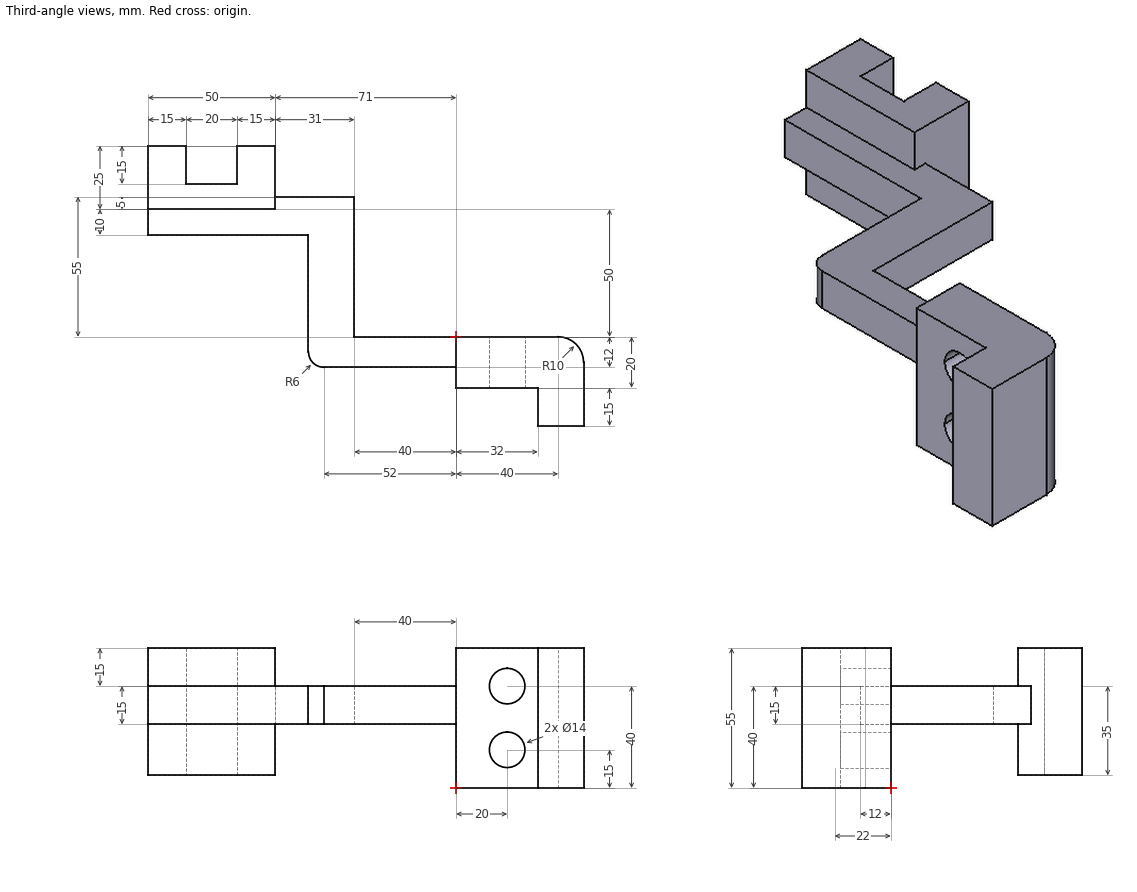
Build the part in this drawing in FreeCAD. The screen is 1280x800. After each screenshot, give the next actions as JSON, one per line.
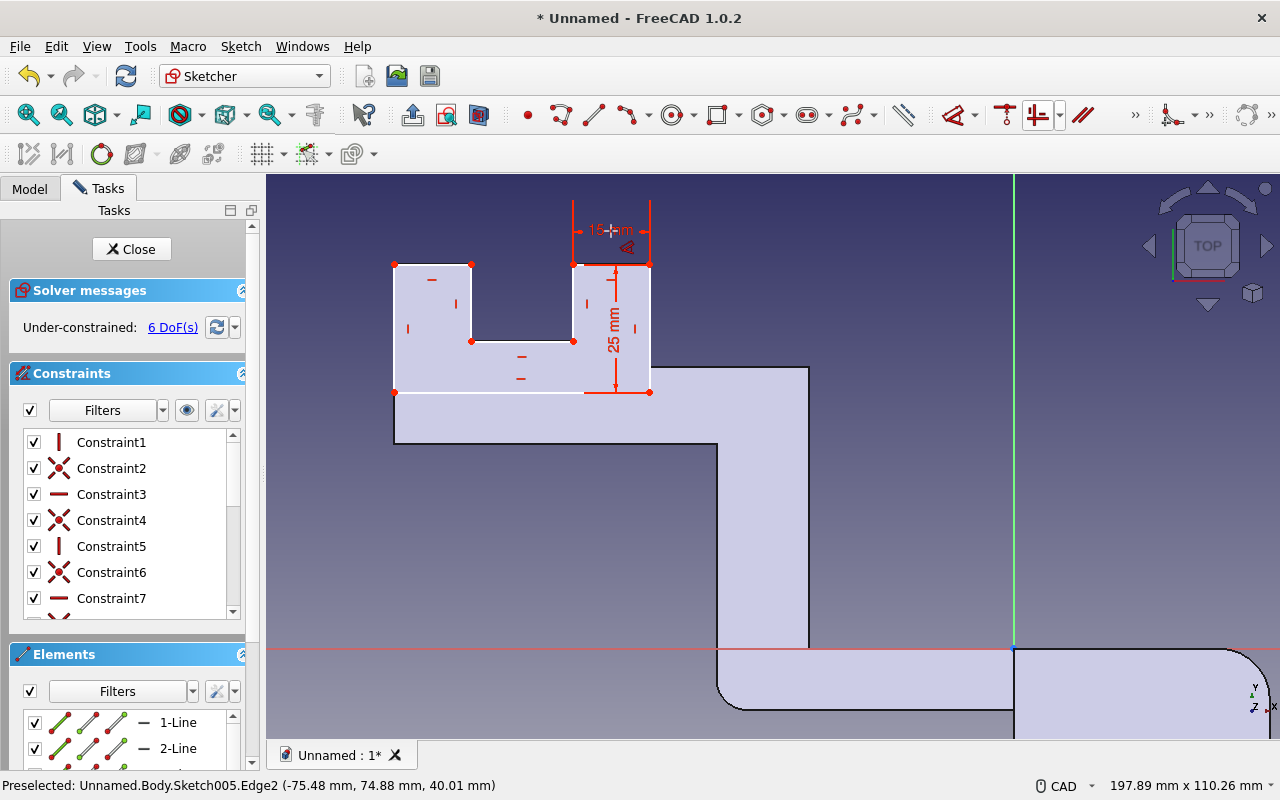
{"action": "left_click", "coordinate": [573, 288]}
{"action": "left_click", "coordinate": [539, 303]}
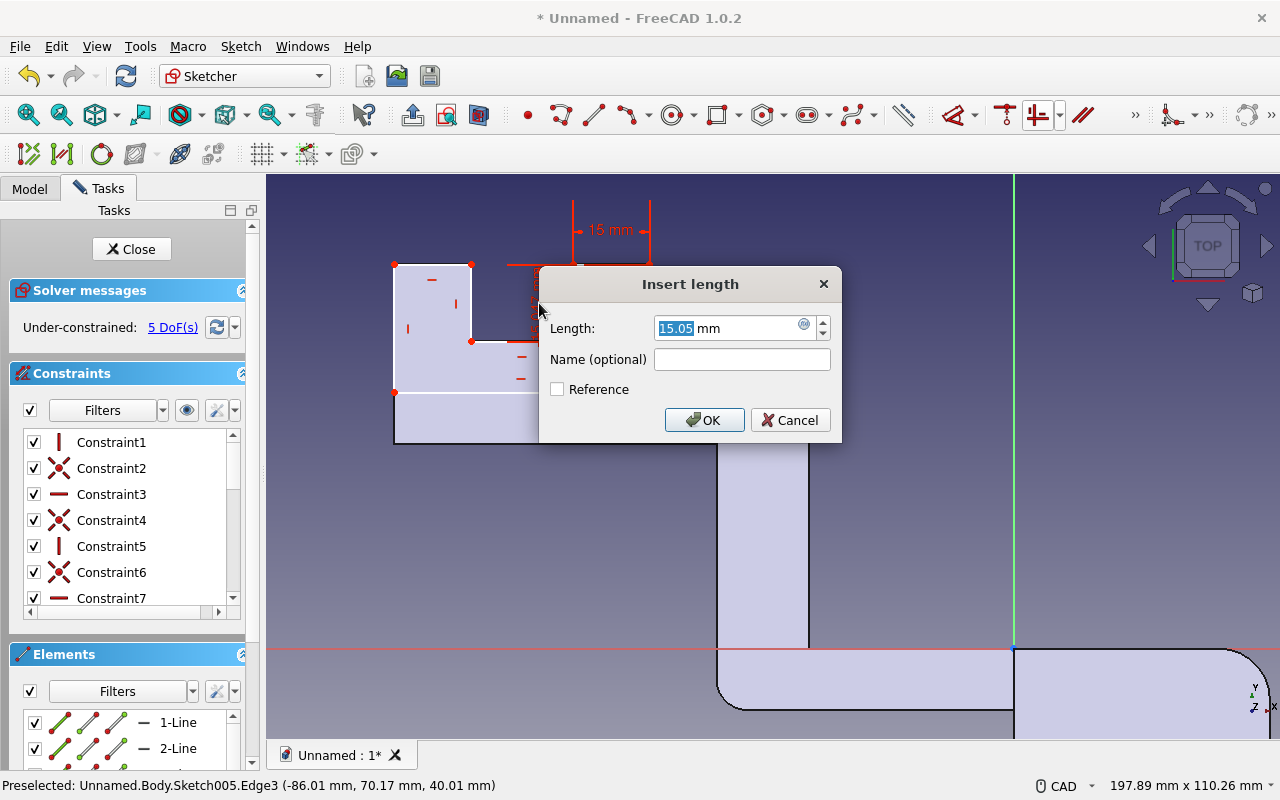
{"action": "type", "text": "15"}
{"action": "key", "text": "Return"}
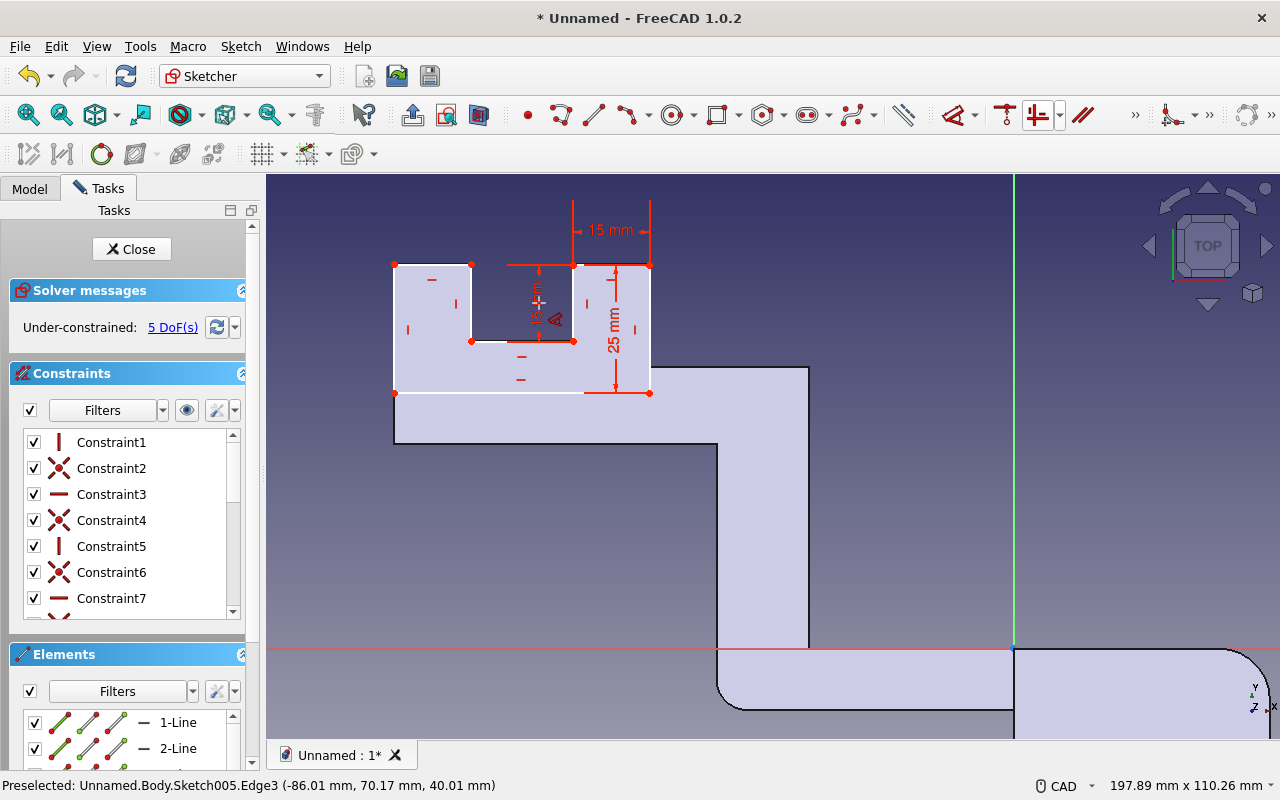
{"action": "left_click", "coordinate": [542, 342]}
{"action": "left_click", "coordinate": [522, 376]}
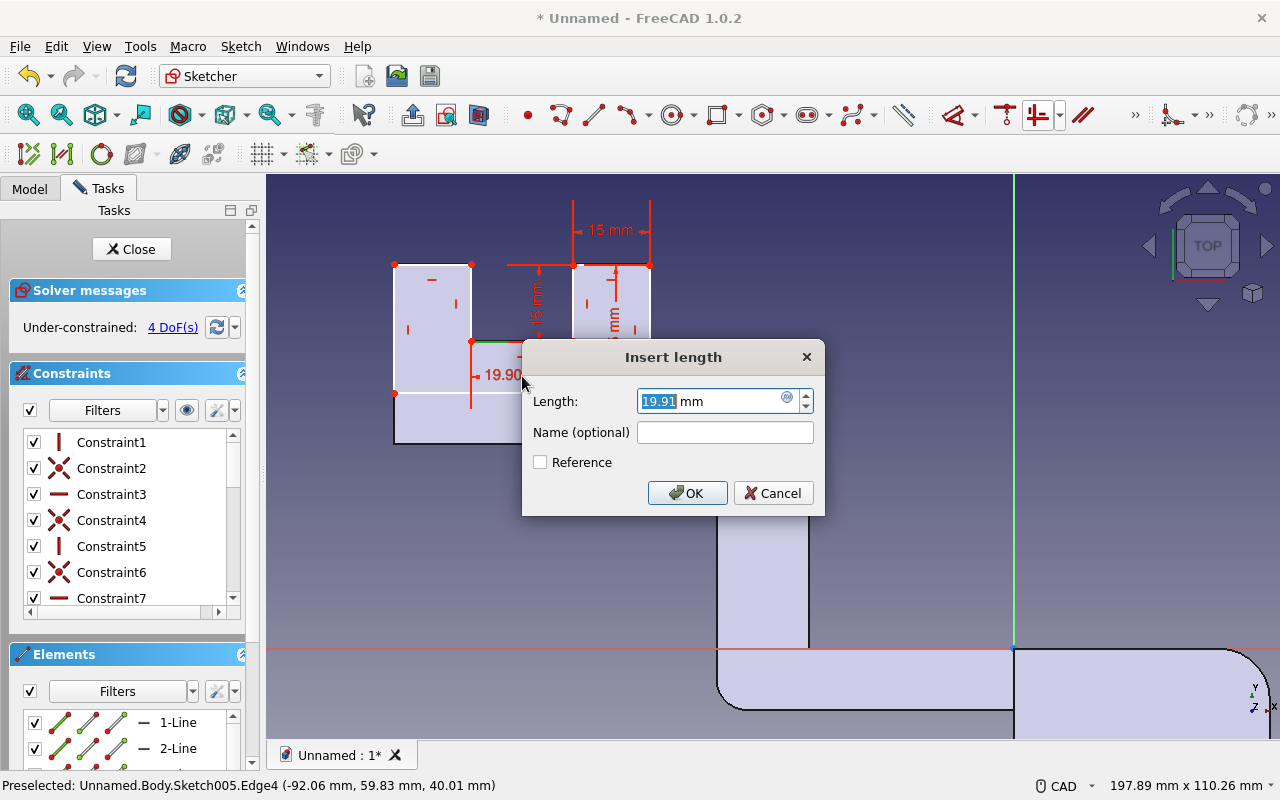
{"action": "type", "text": "20"}
{"action": "key", "text": "Return"}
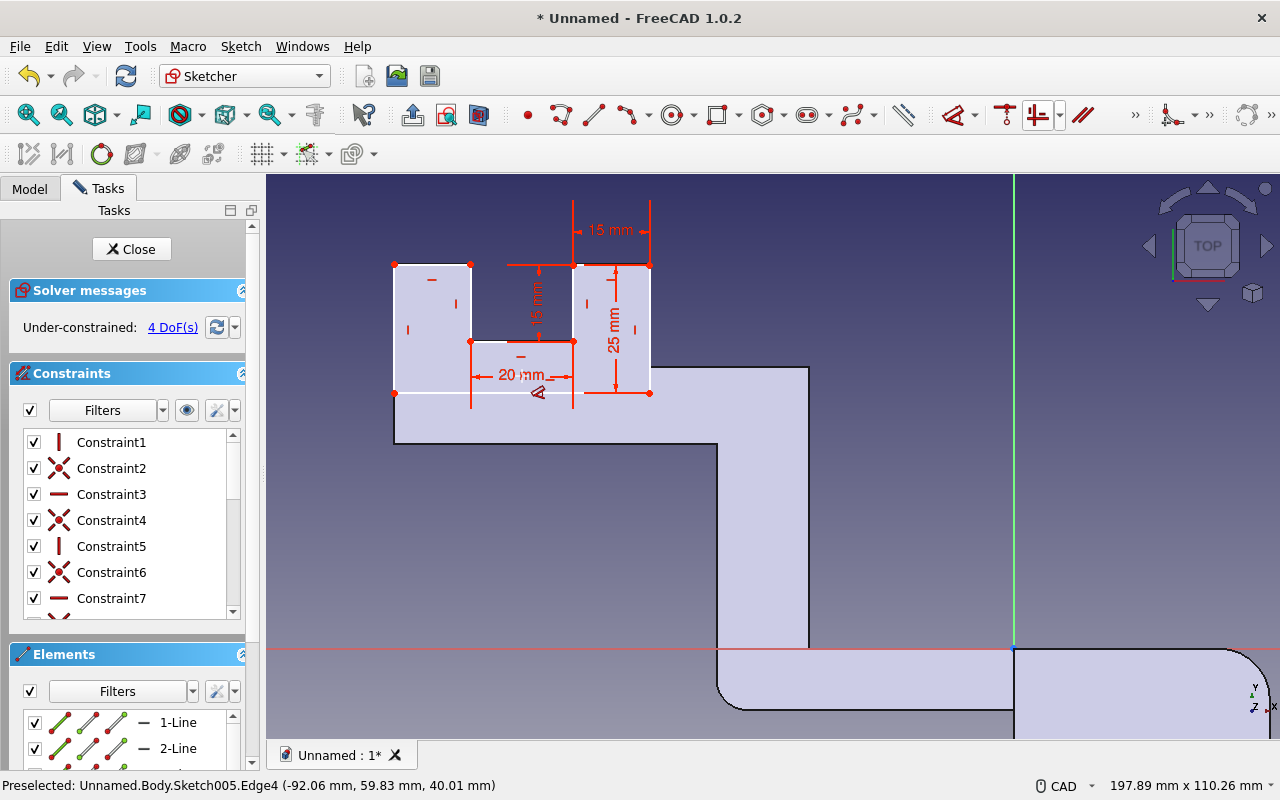
{"action": "left_click", "coordinate": [471, 319]}
{"action": "left_click", "coordinate": [437, 304]}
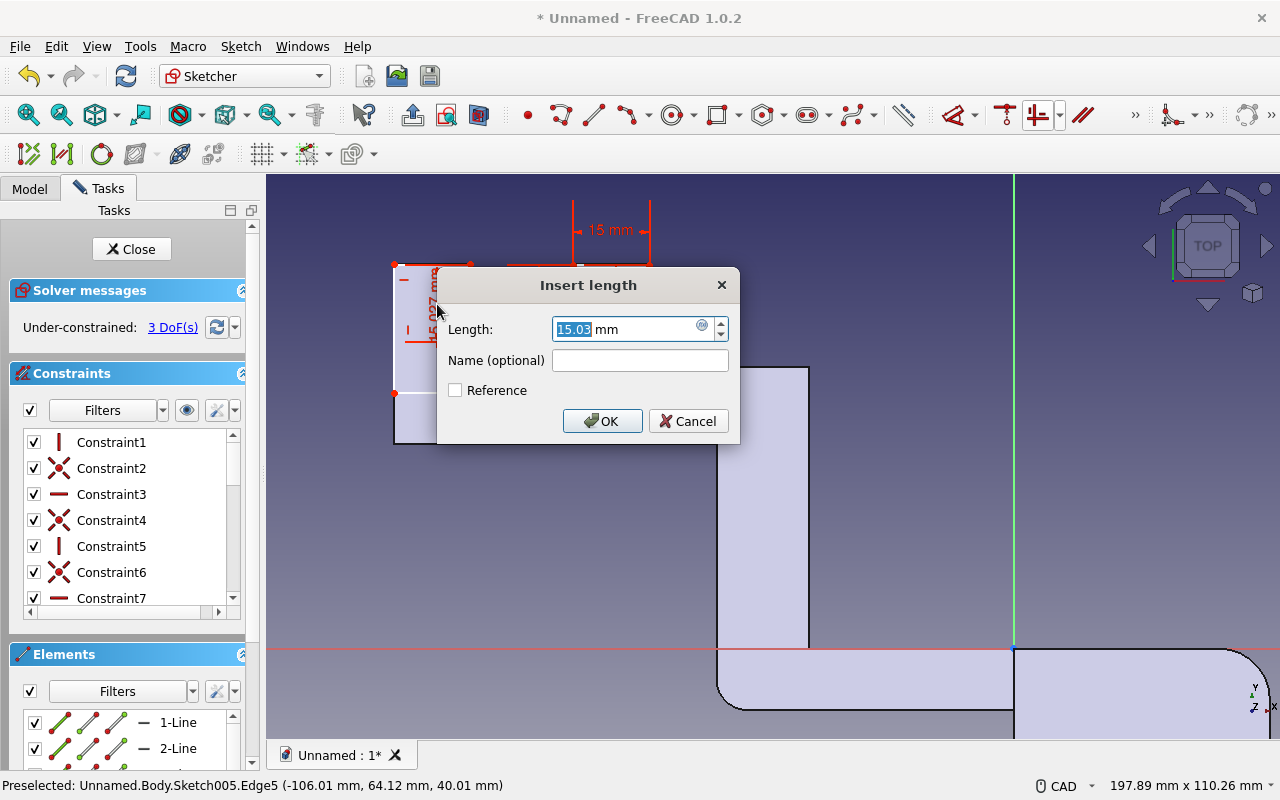
{"action": "type", "text": "15"}
{"action": "key", "text": "Return"}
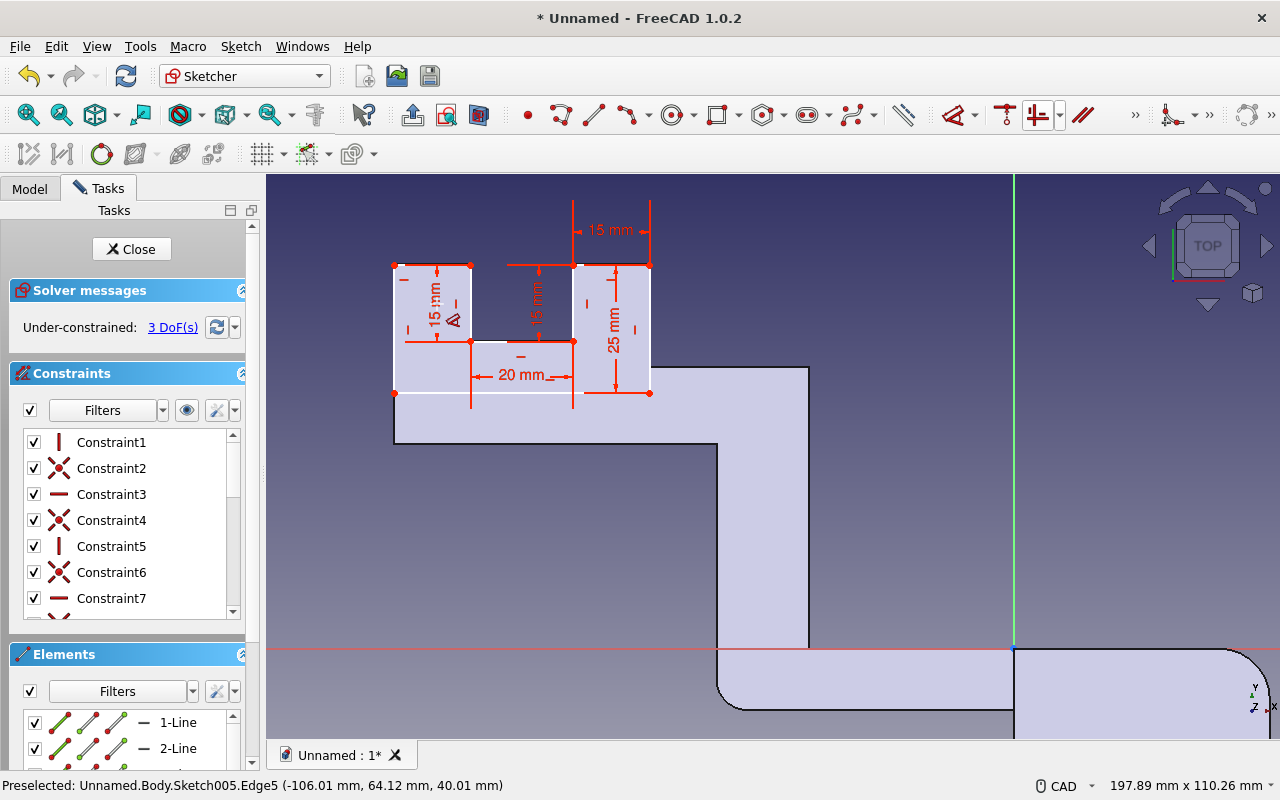
{"action": "left_click", "coordinate": [448, 265]}
{"action": "left_click", "coordinate": [432, 231]}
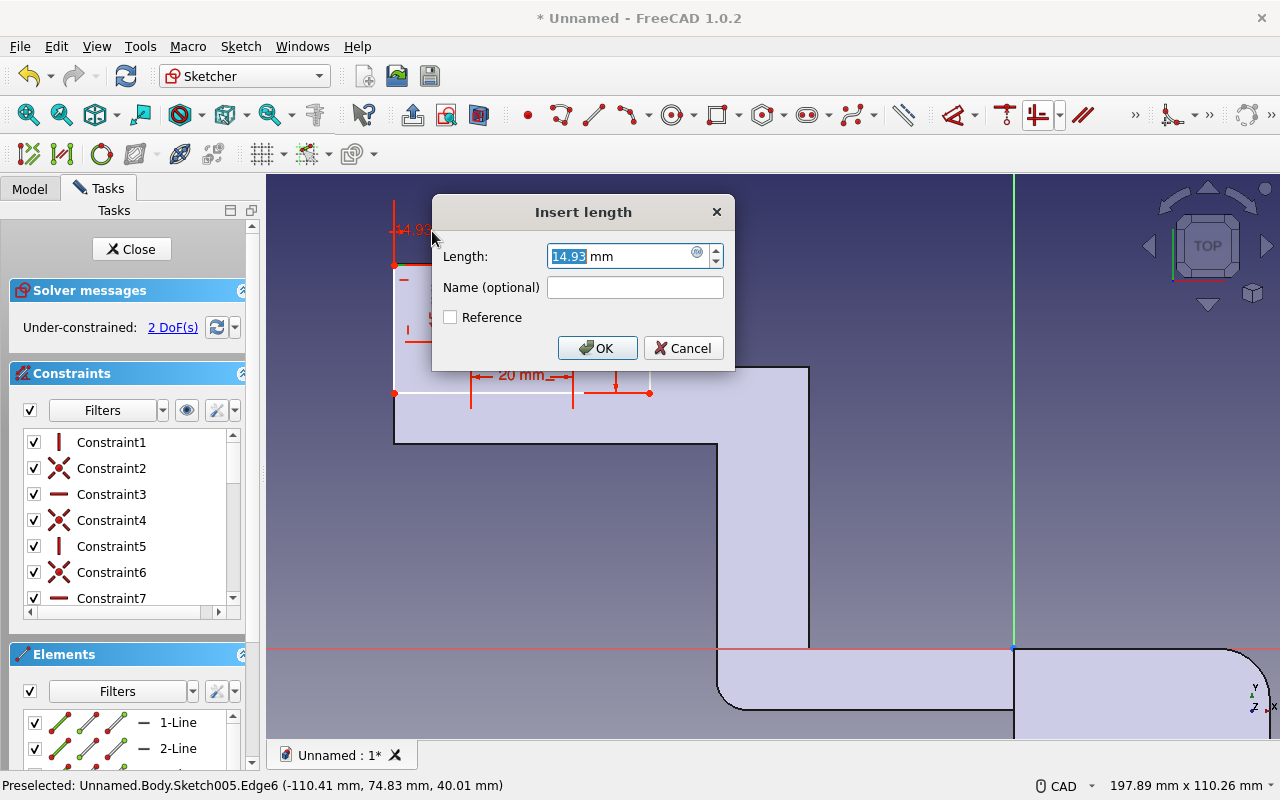
{"action": "type", "text": "15"}
{"action": "key", "text": "Return"}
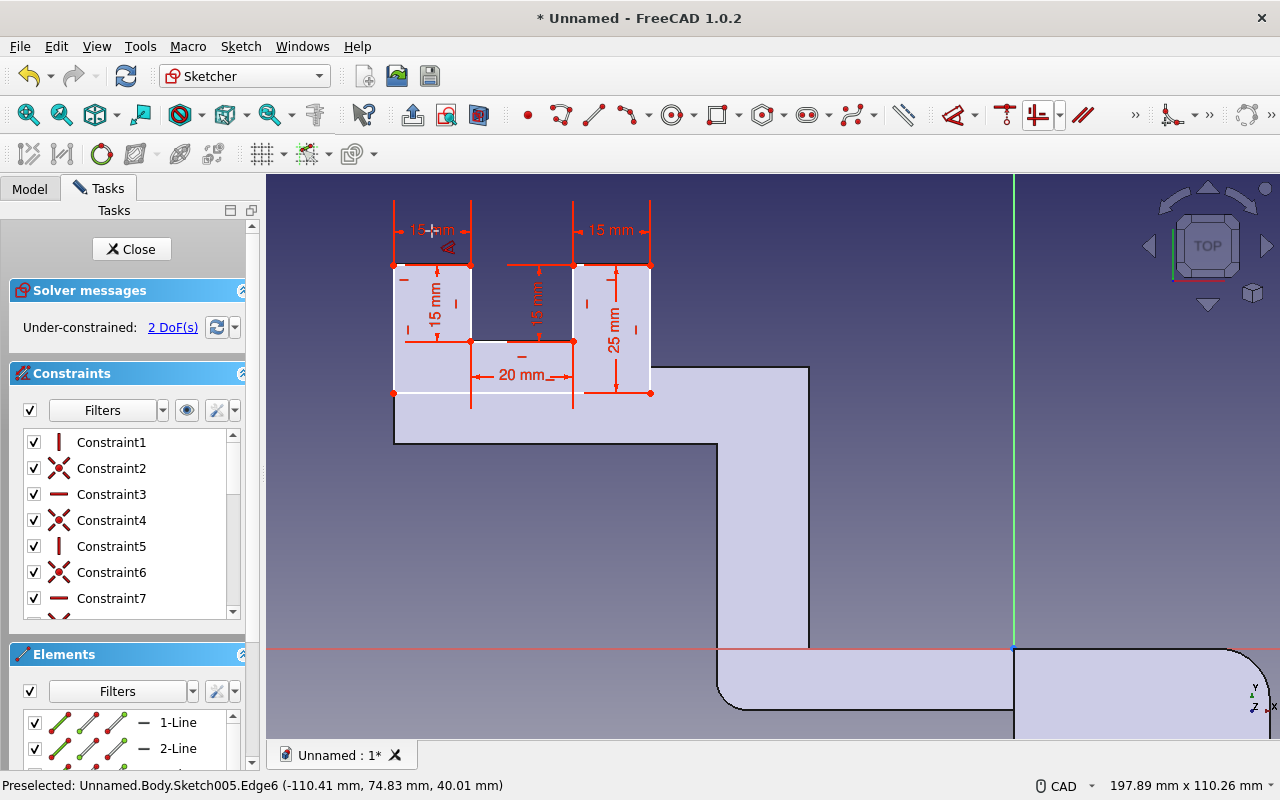
{"action": "left_click", "coordinate": [650, 393]}
{"action": "left_click", "coordinate": [832, 683]}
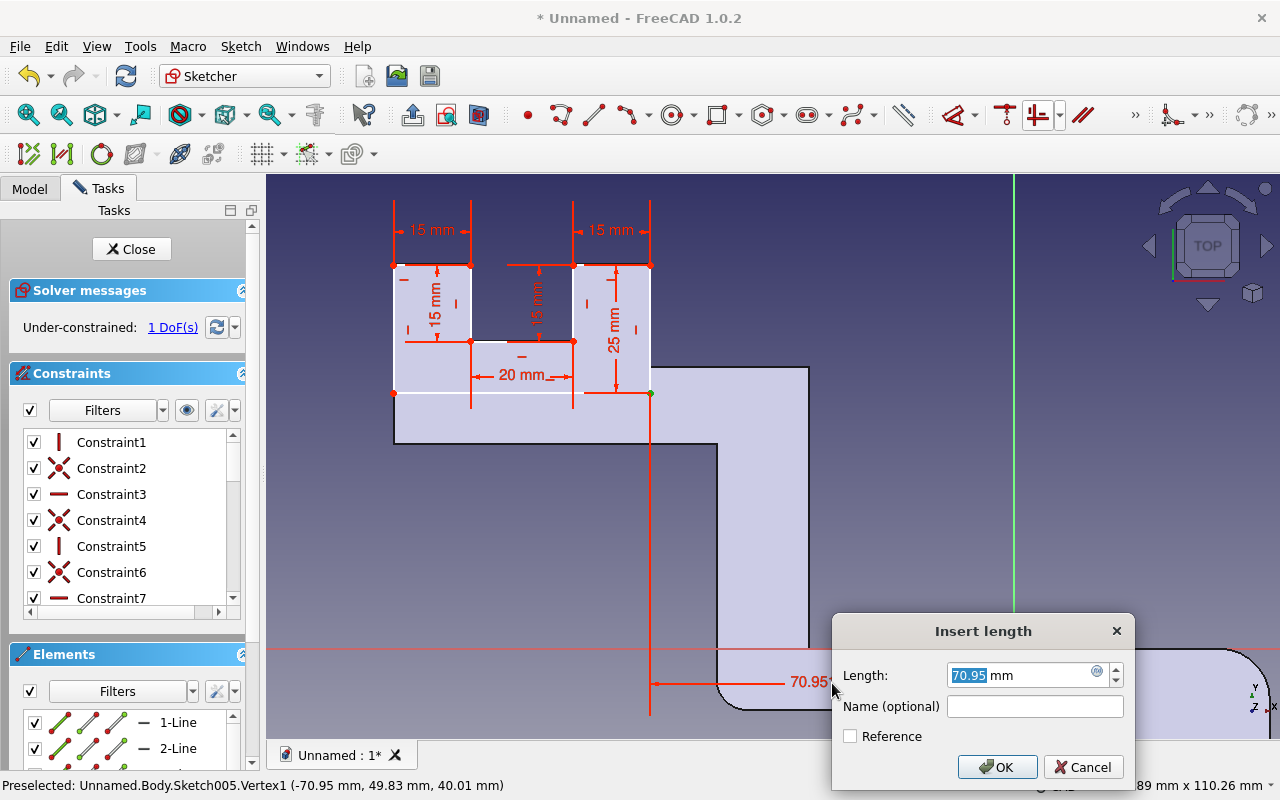
{"action": "type", "text": "71"}
{"action": "key", "text": "Return"}